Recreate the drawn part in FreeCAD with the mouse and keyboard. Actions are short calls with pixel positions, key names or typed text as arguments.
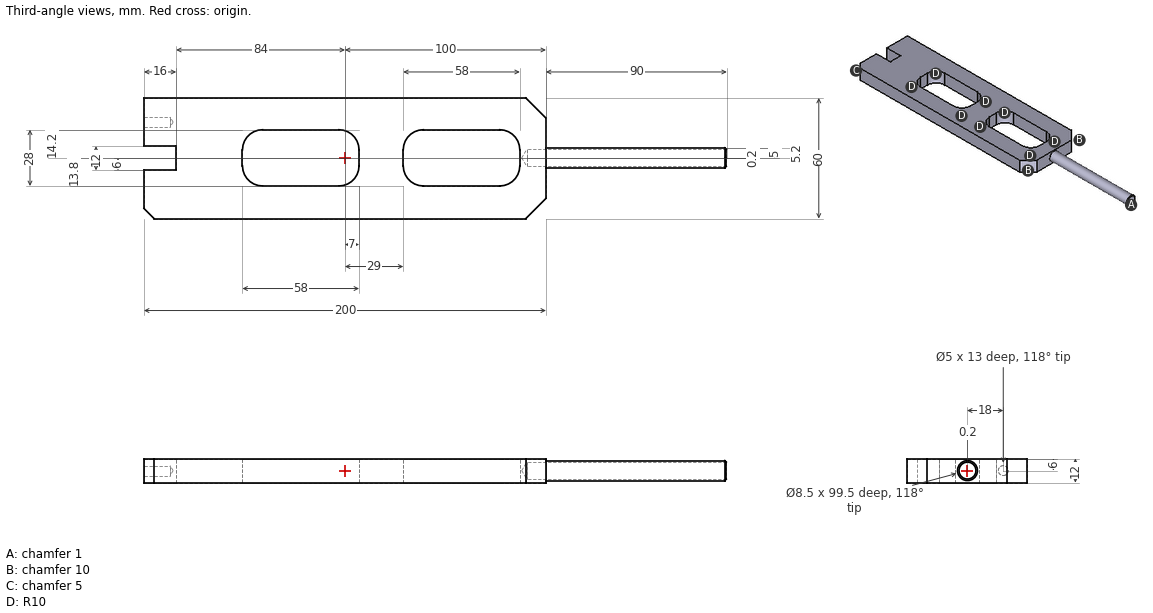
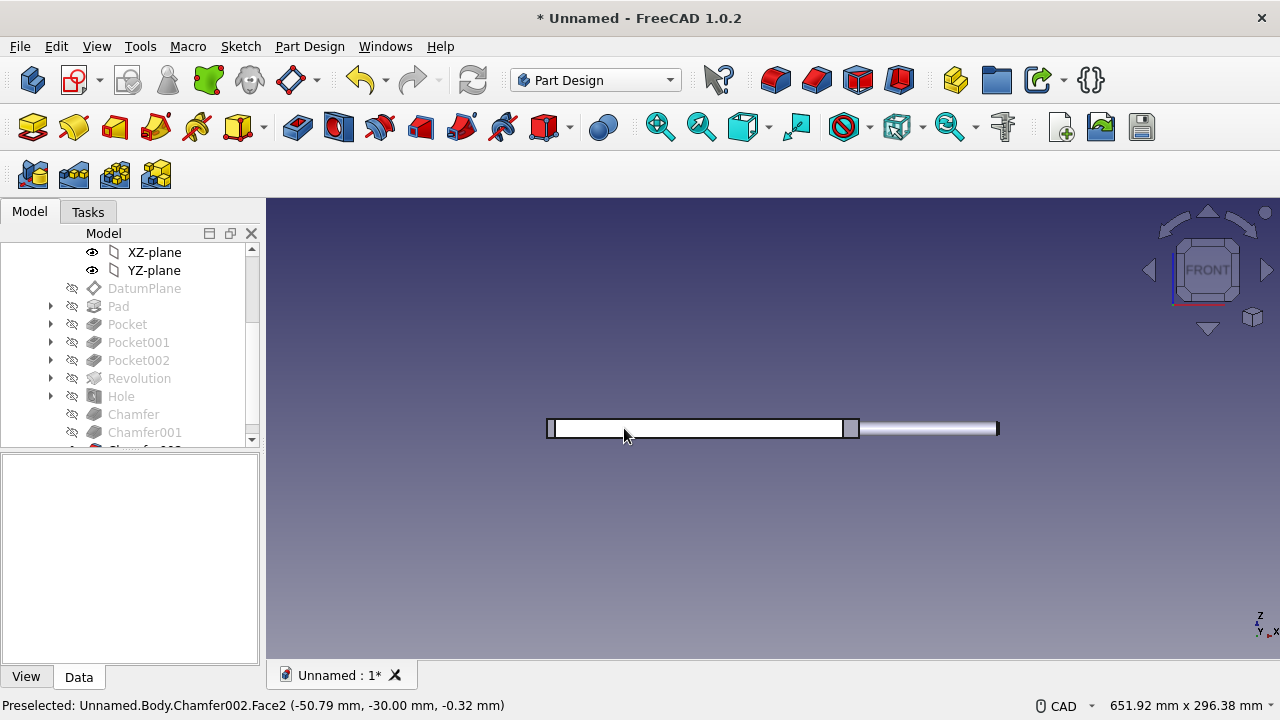
key(3)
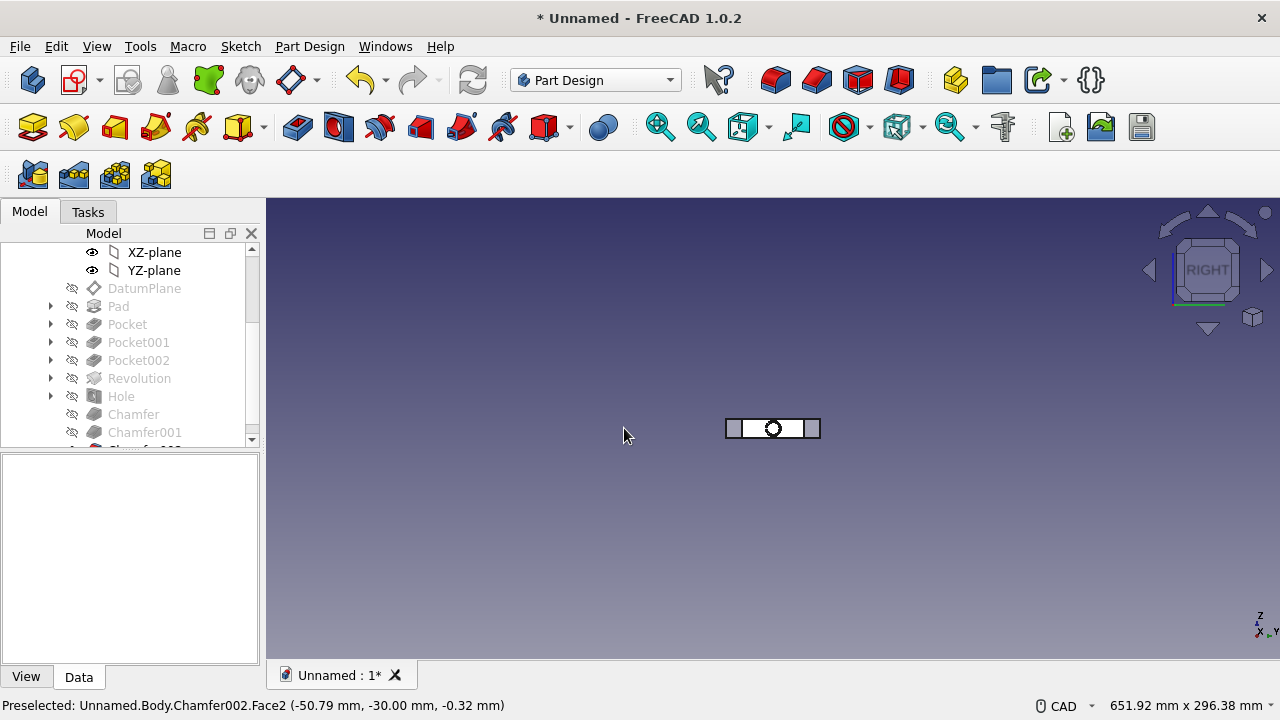
click(661, 128)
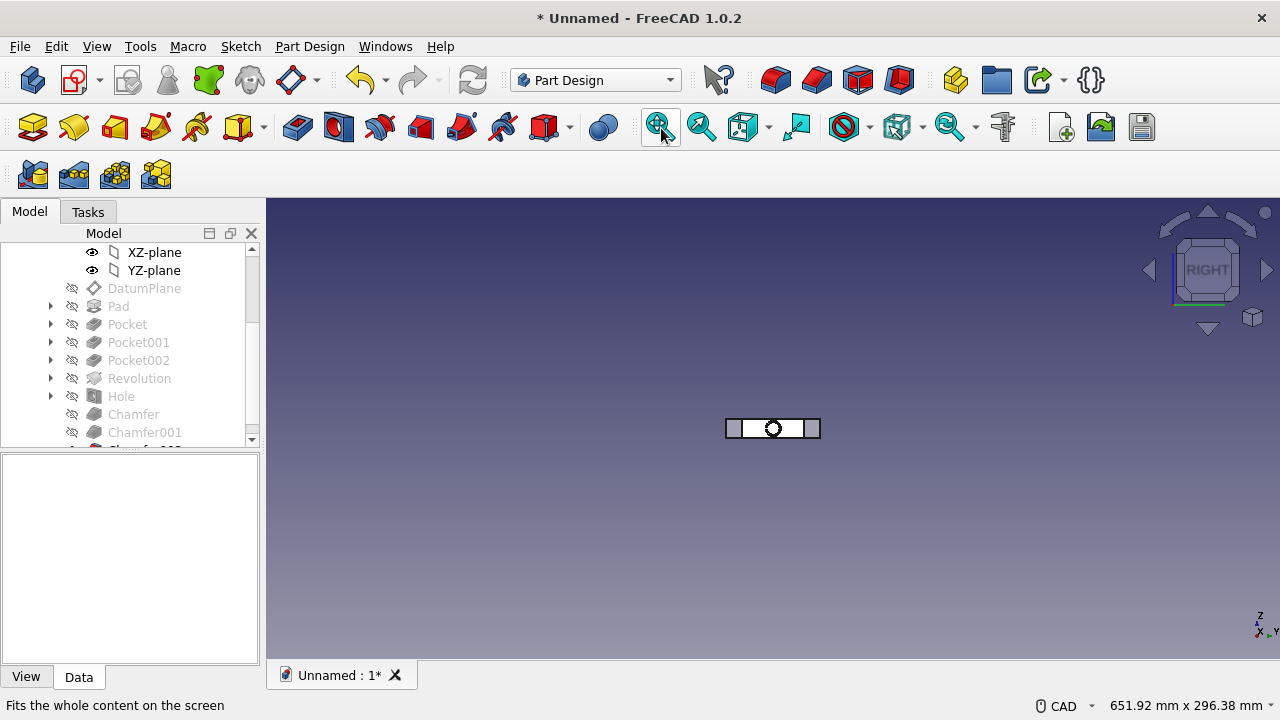
scroll(752, 427, up, 4)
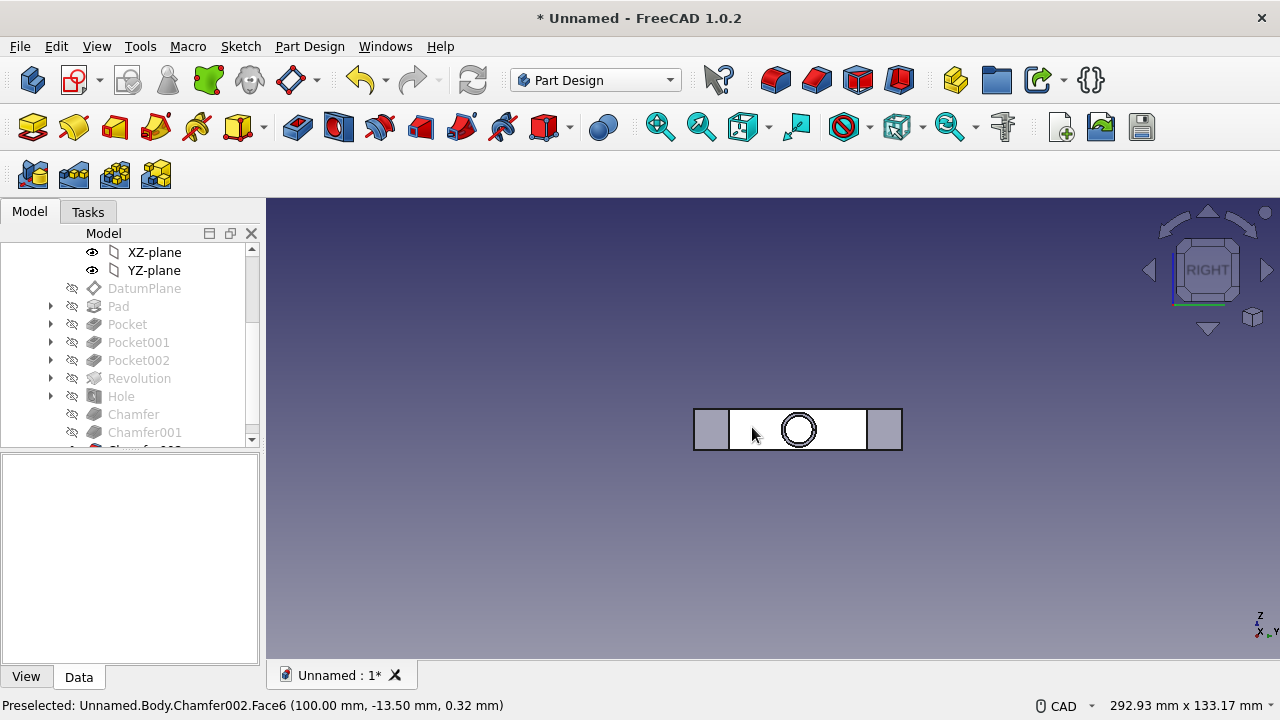
key(v)
key(f)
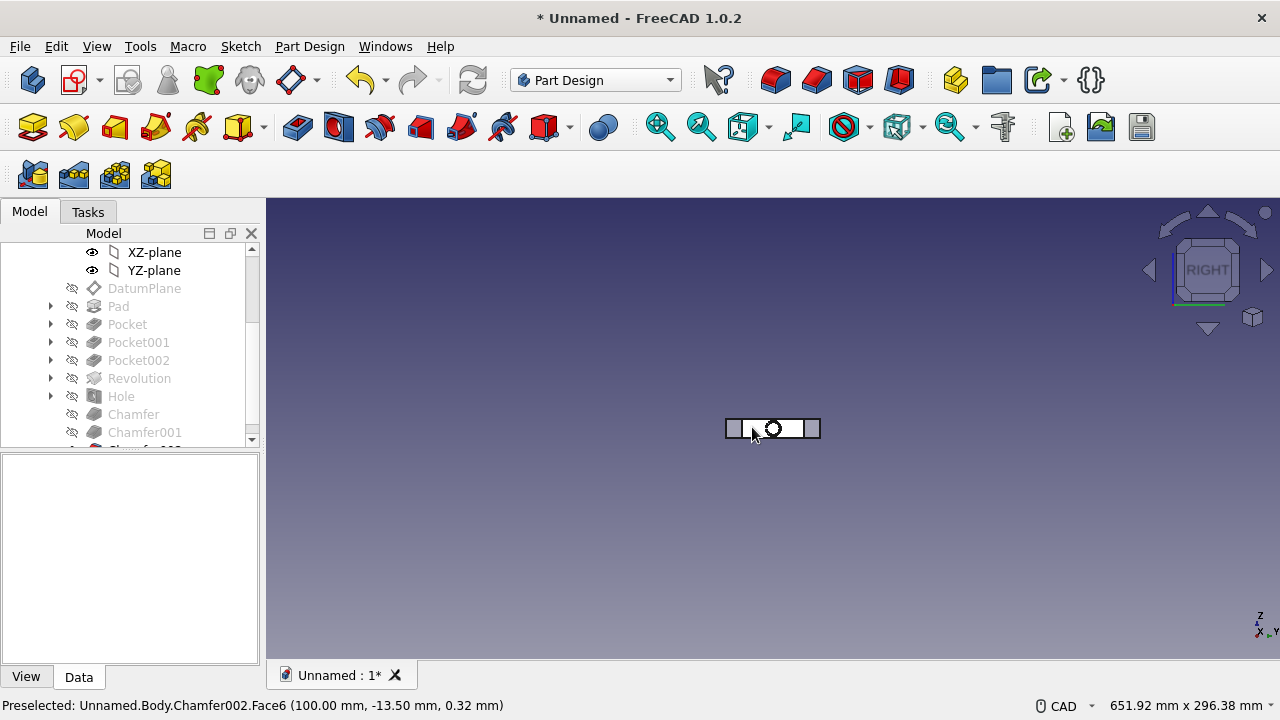
key(5)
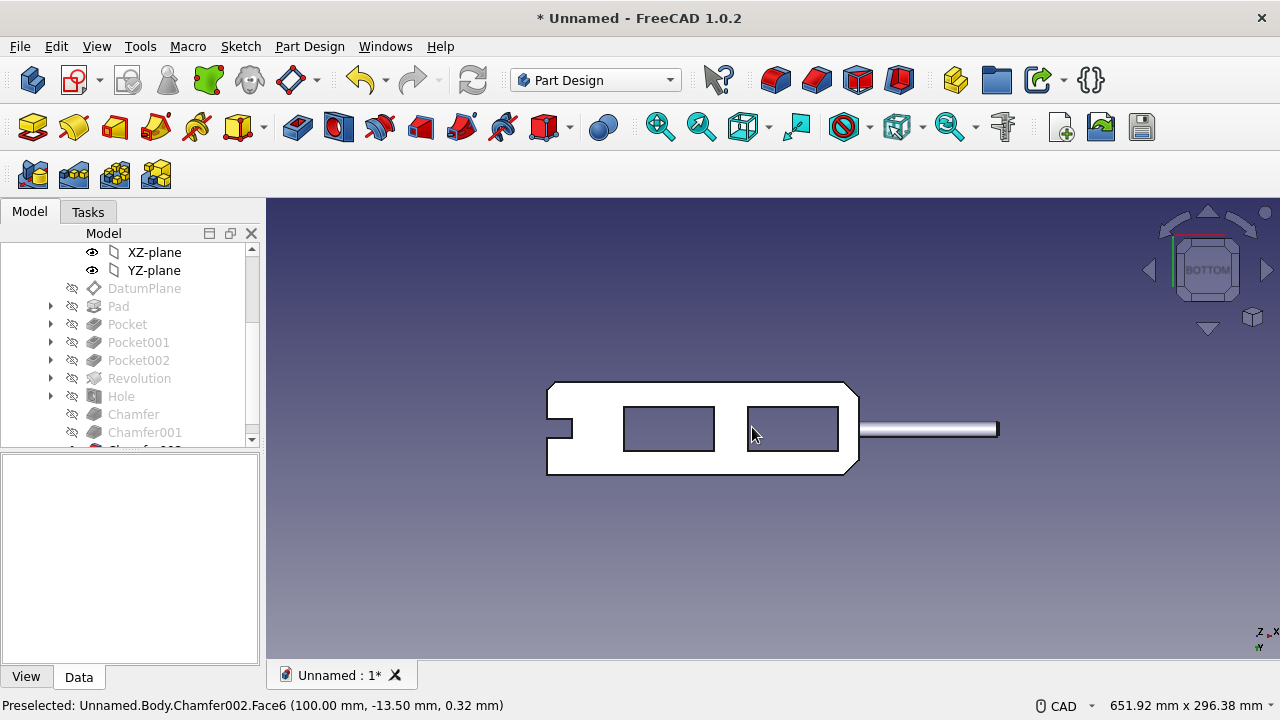
key(v)
key(f)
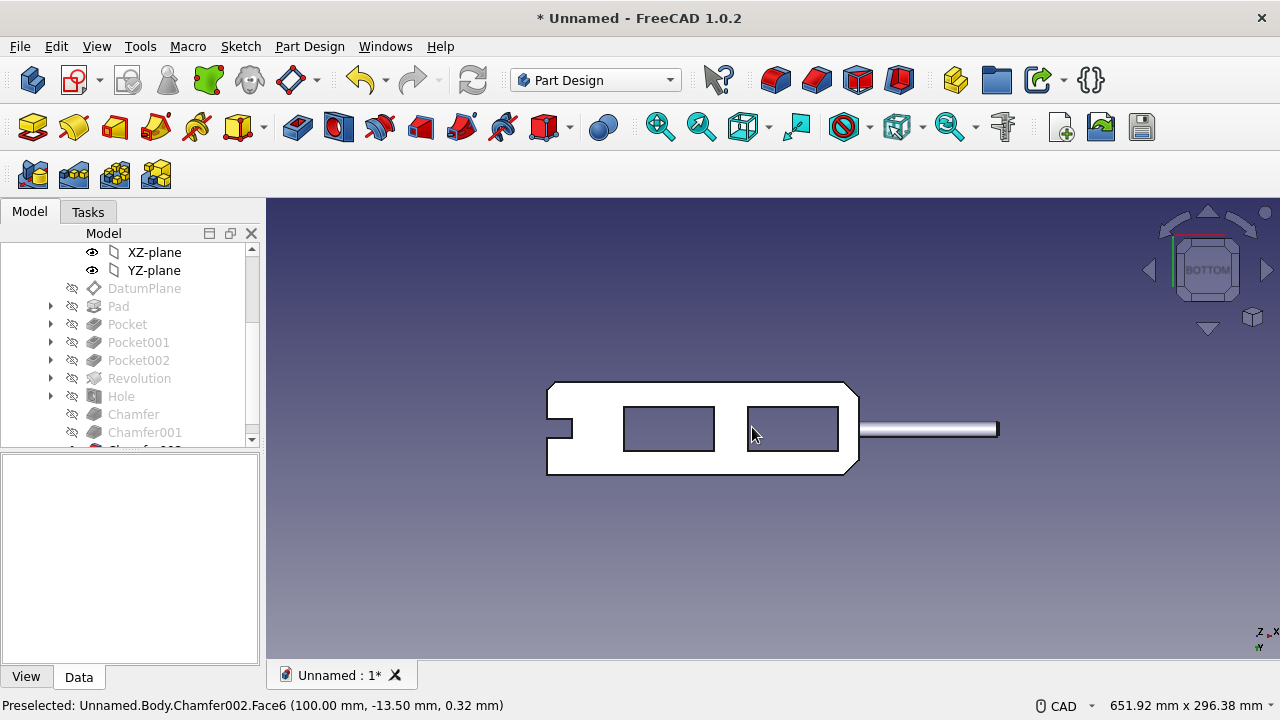
scroll(624, 406, up, 4)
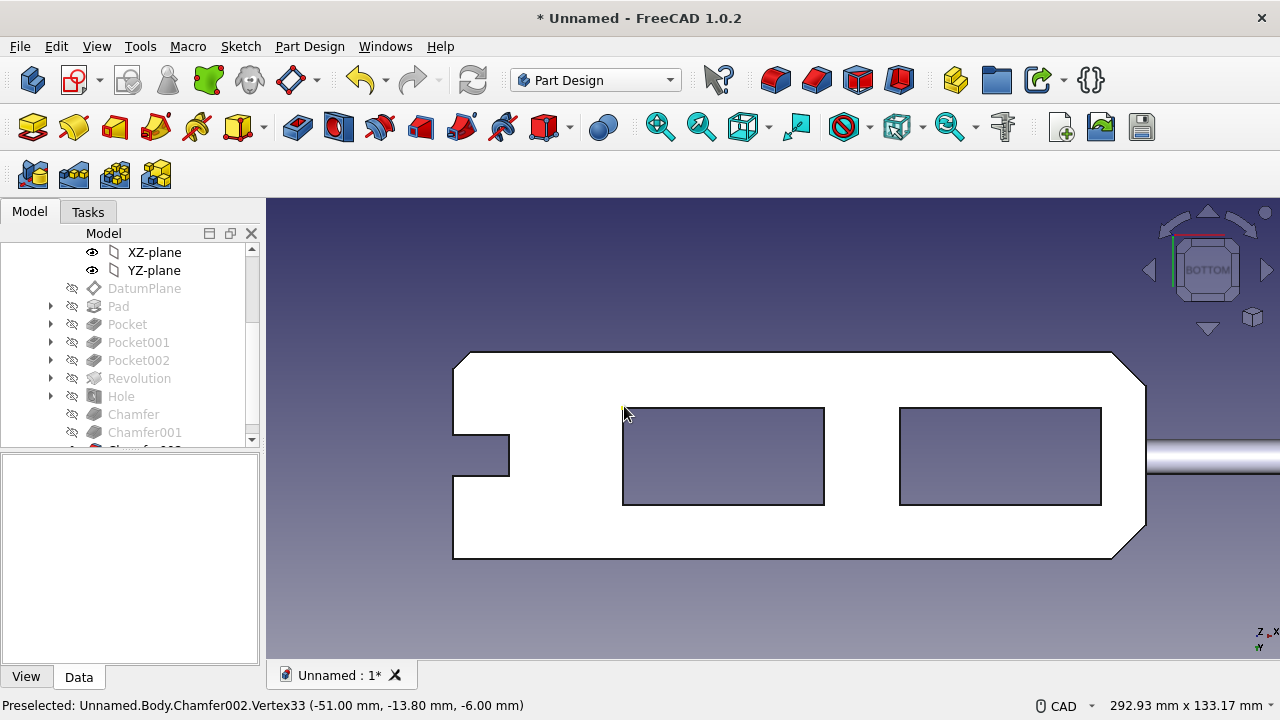
key(v)
key(f)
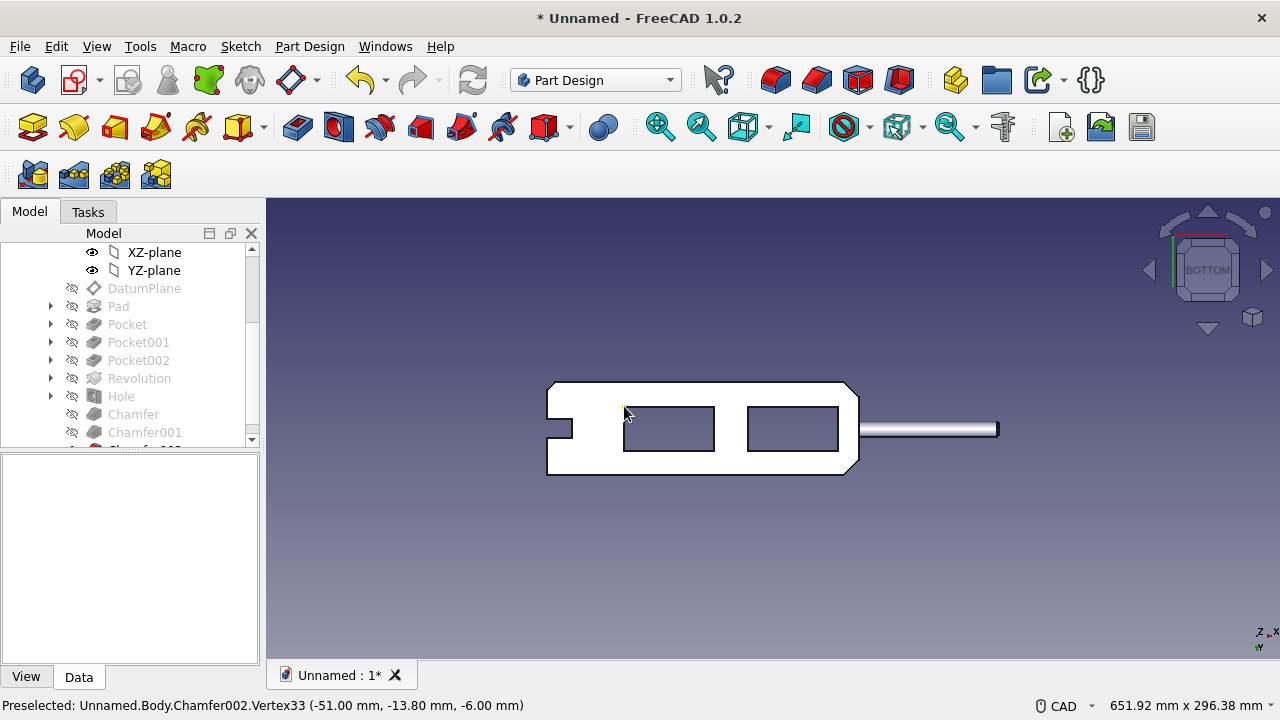
key(4)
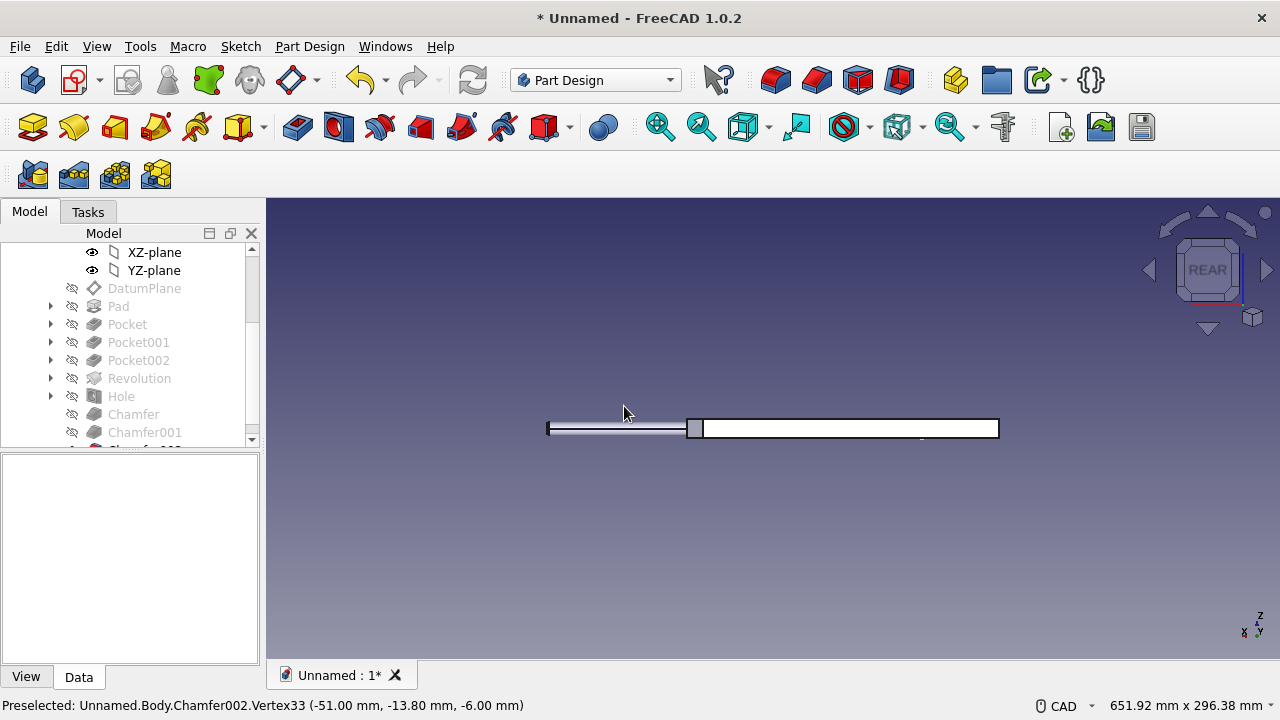
key(v)
key(f)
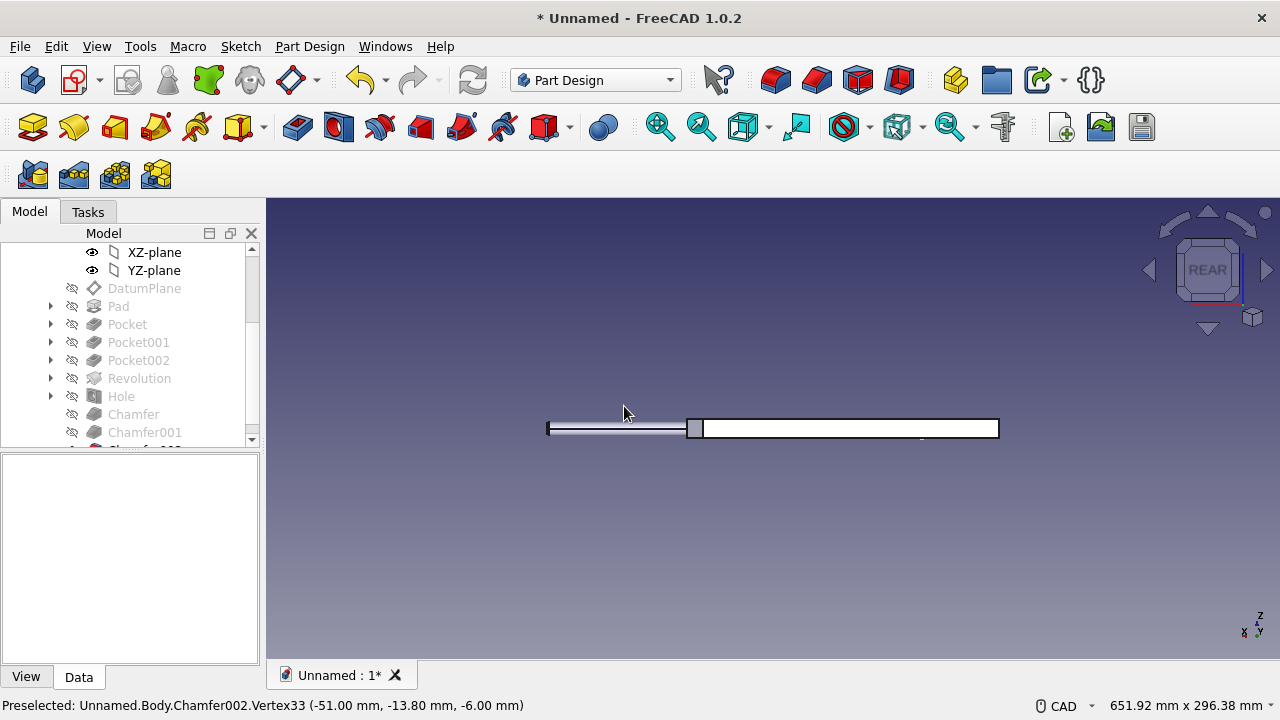
scroll(922, 428, up, 4)